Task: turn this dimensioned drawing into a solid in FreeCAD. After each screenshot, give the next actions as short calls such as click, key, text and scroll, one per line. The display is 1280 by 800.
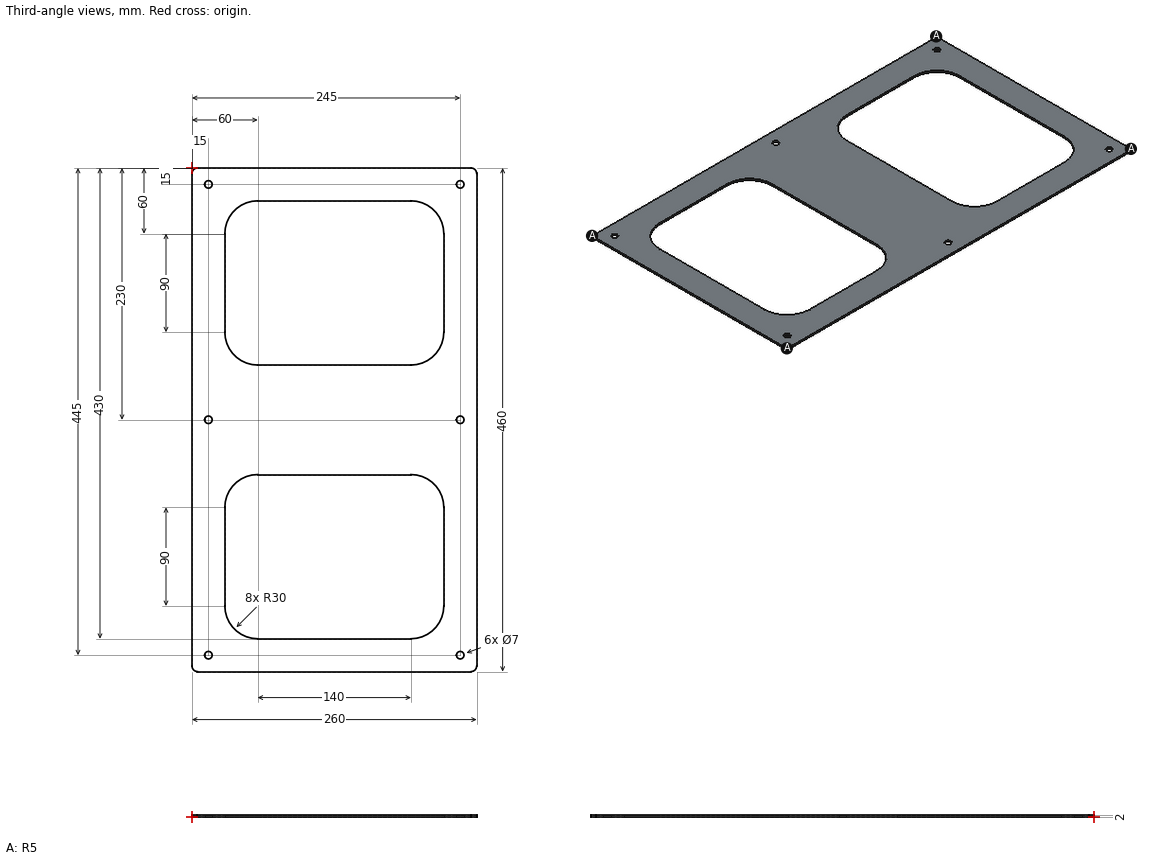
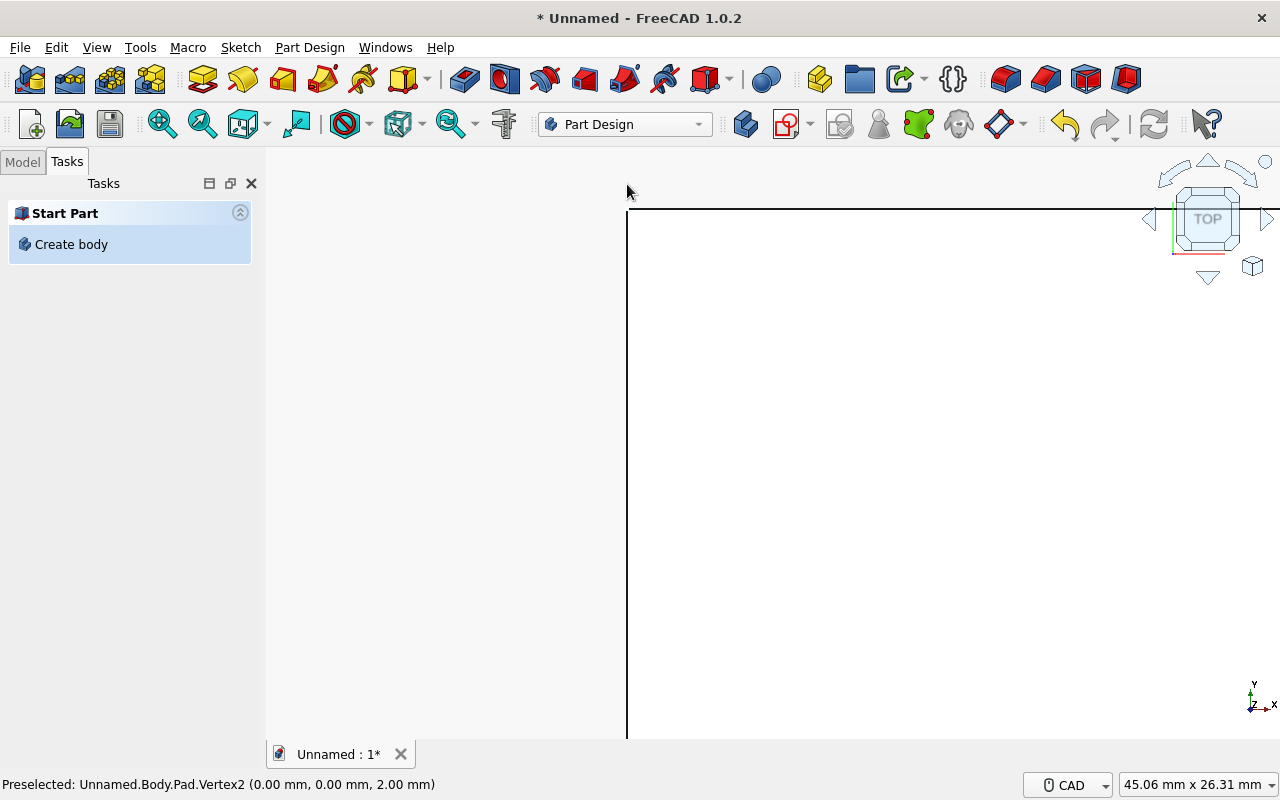
click(164, 124)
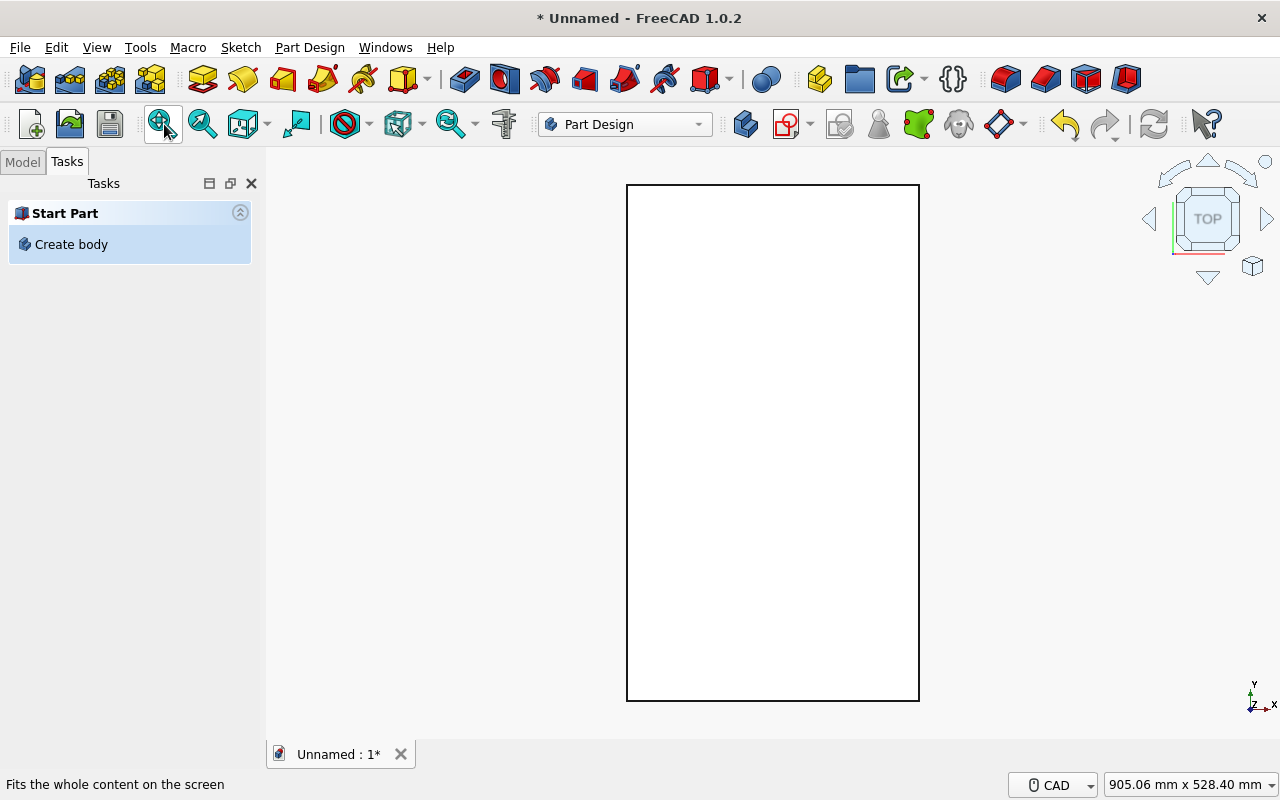
key(1)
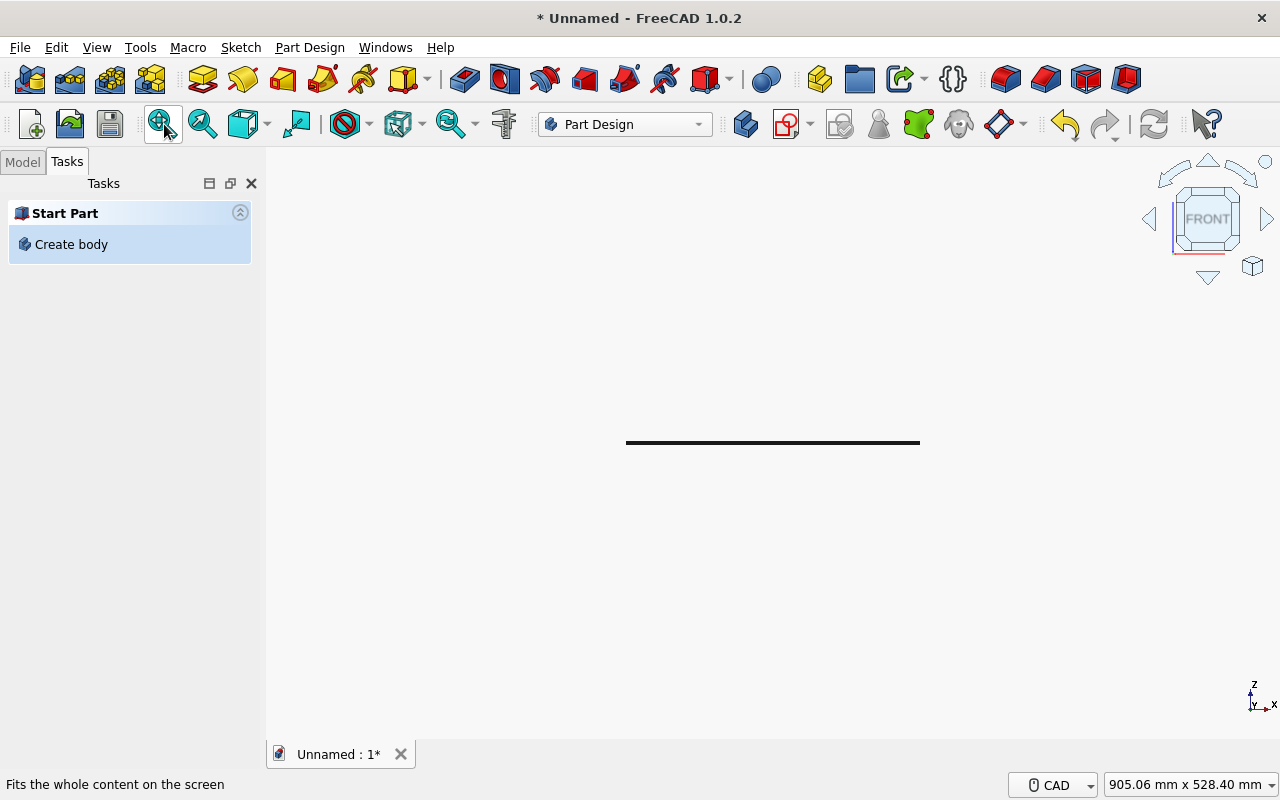
click(164, 124)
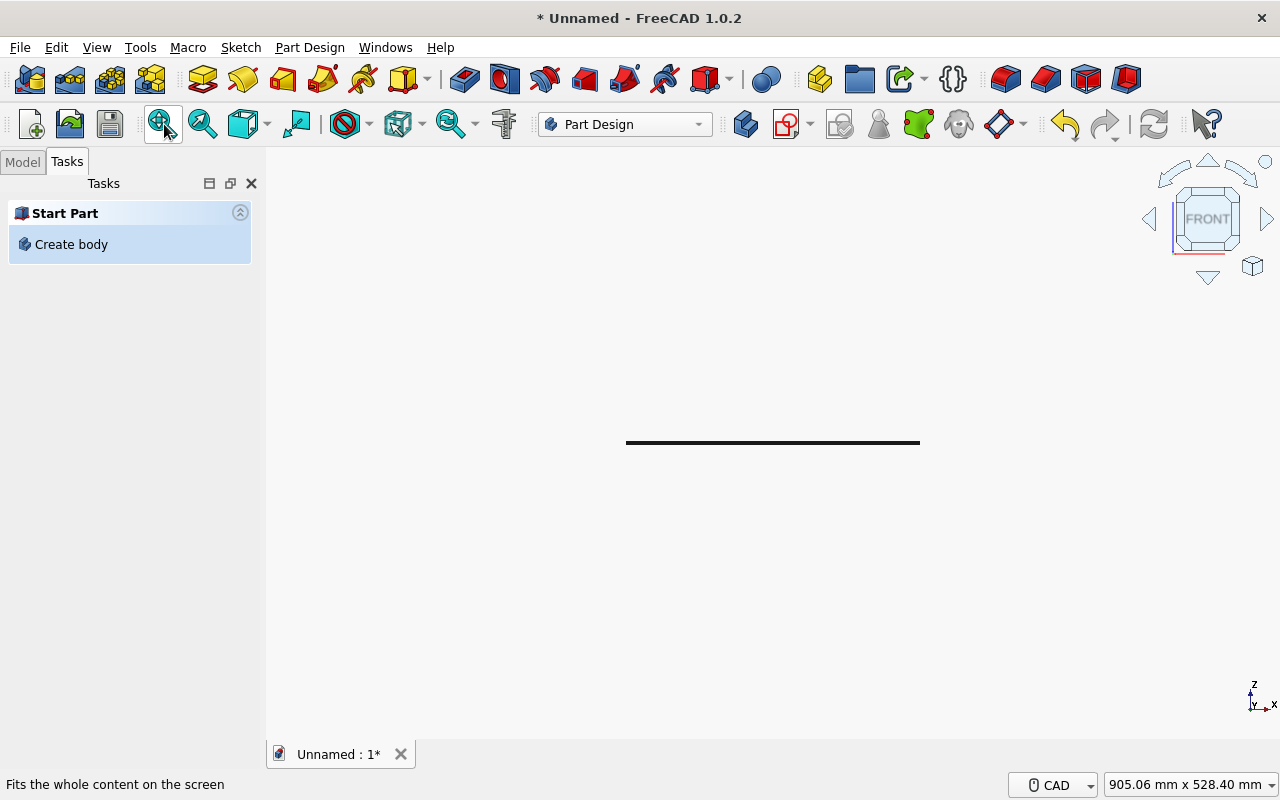
scroll(627, 442, up, 15)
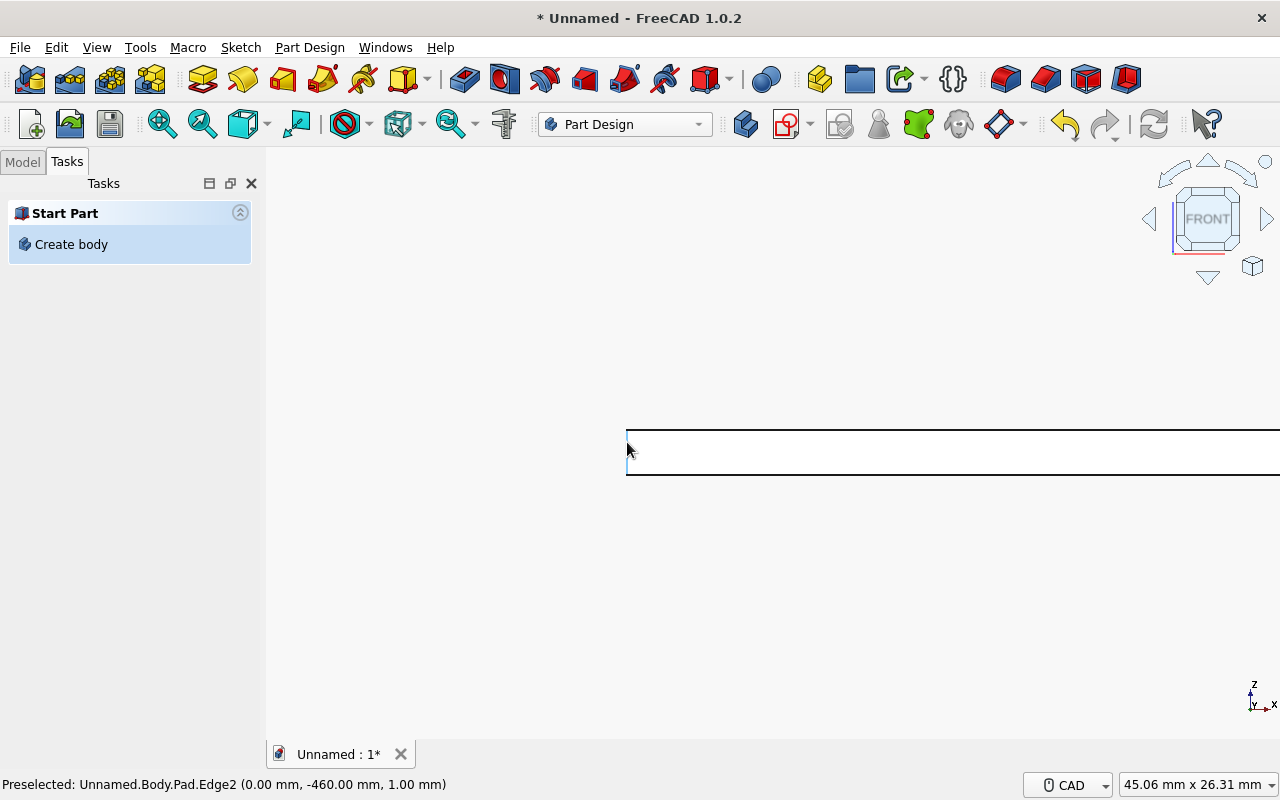
click(627, 452)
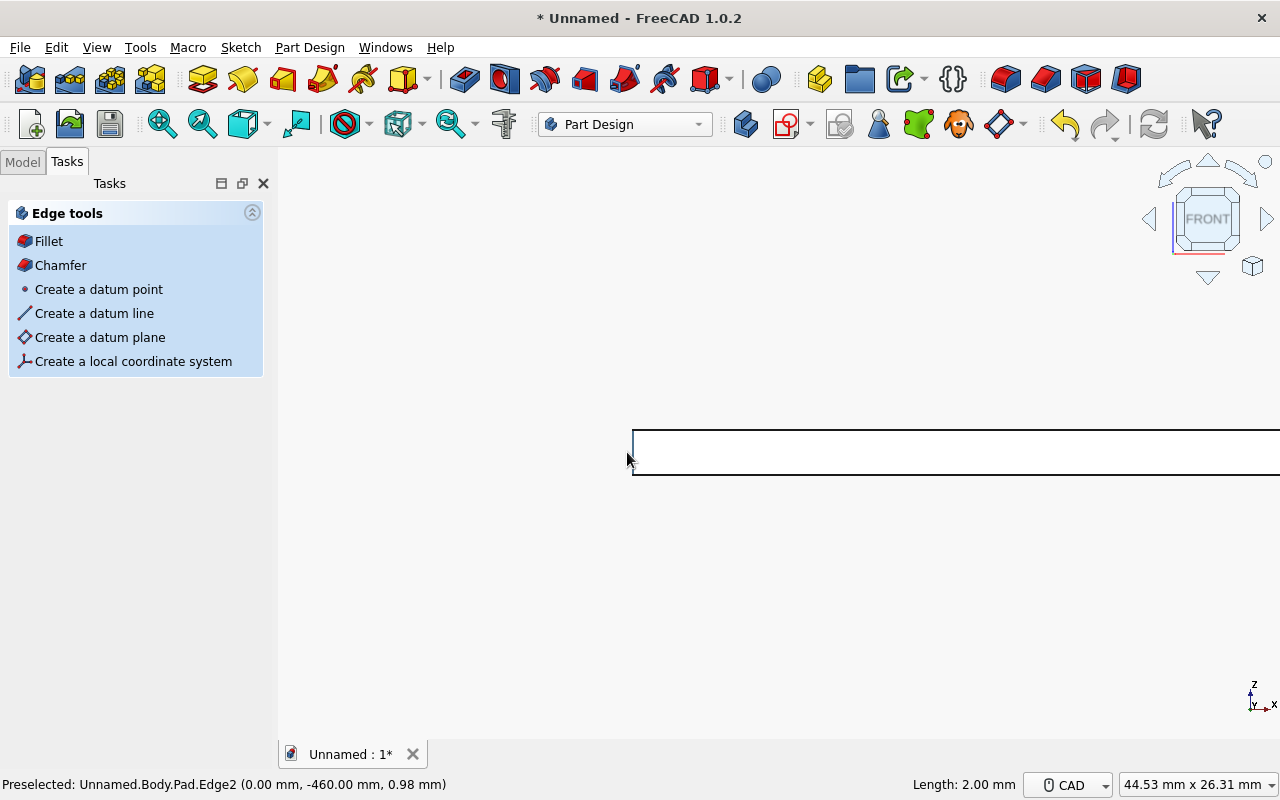
click(164, 124)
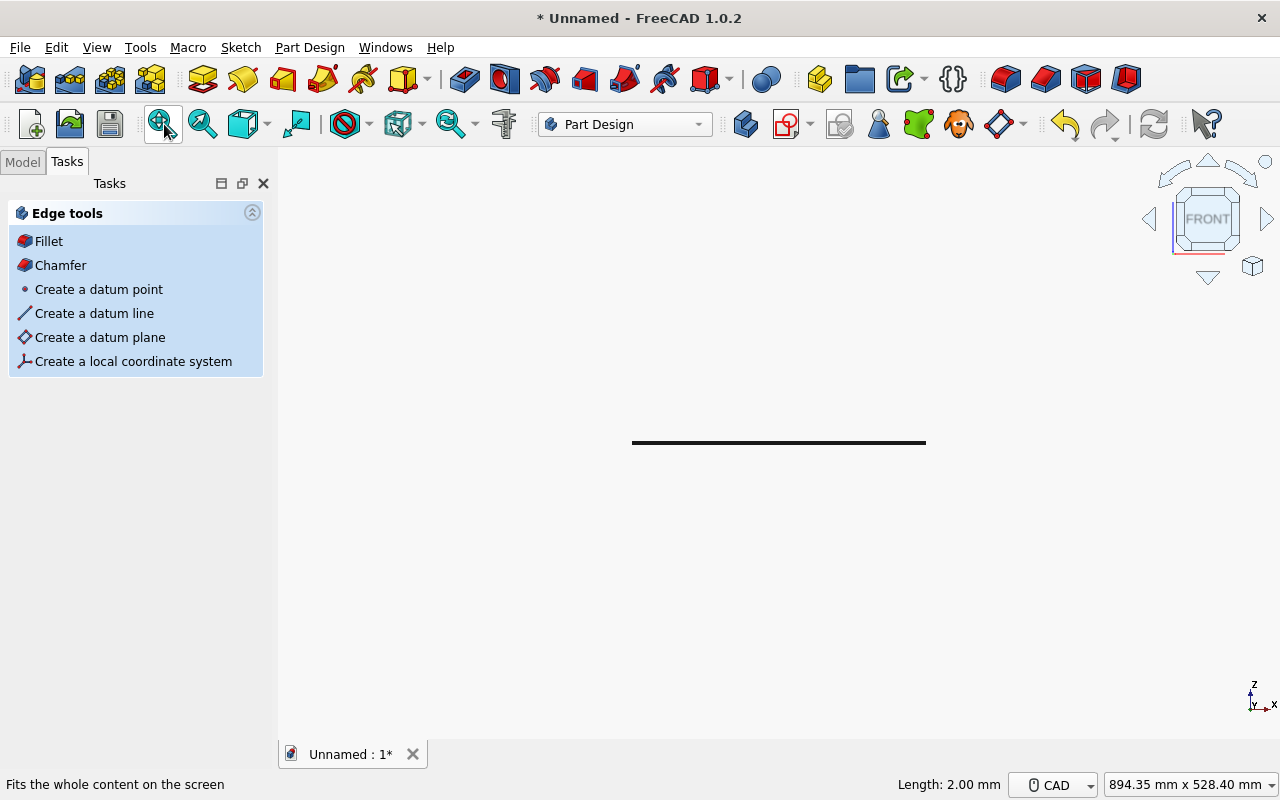
key(3)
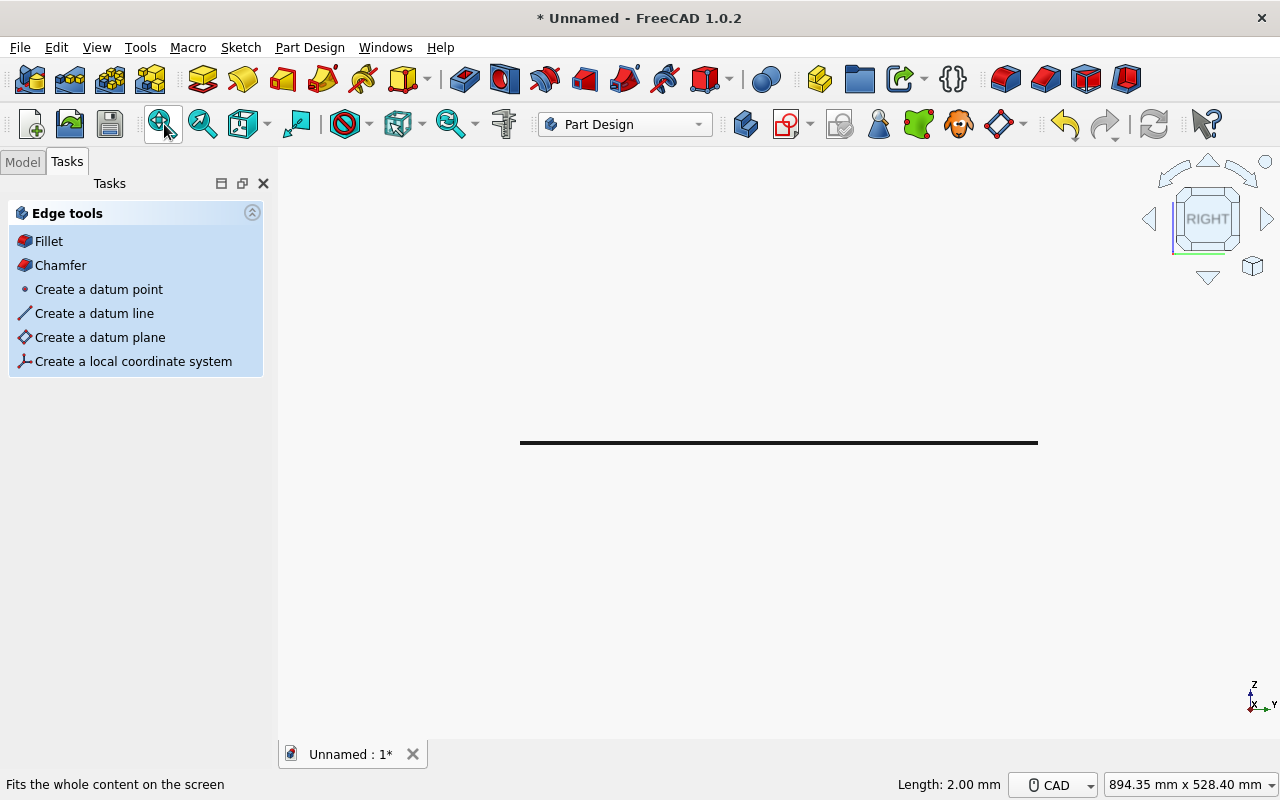
scroll(1037, 442, up, 15)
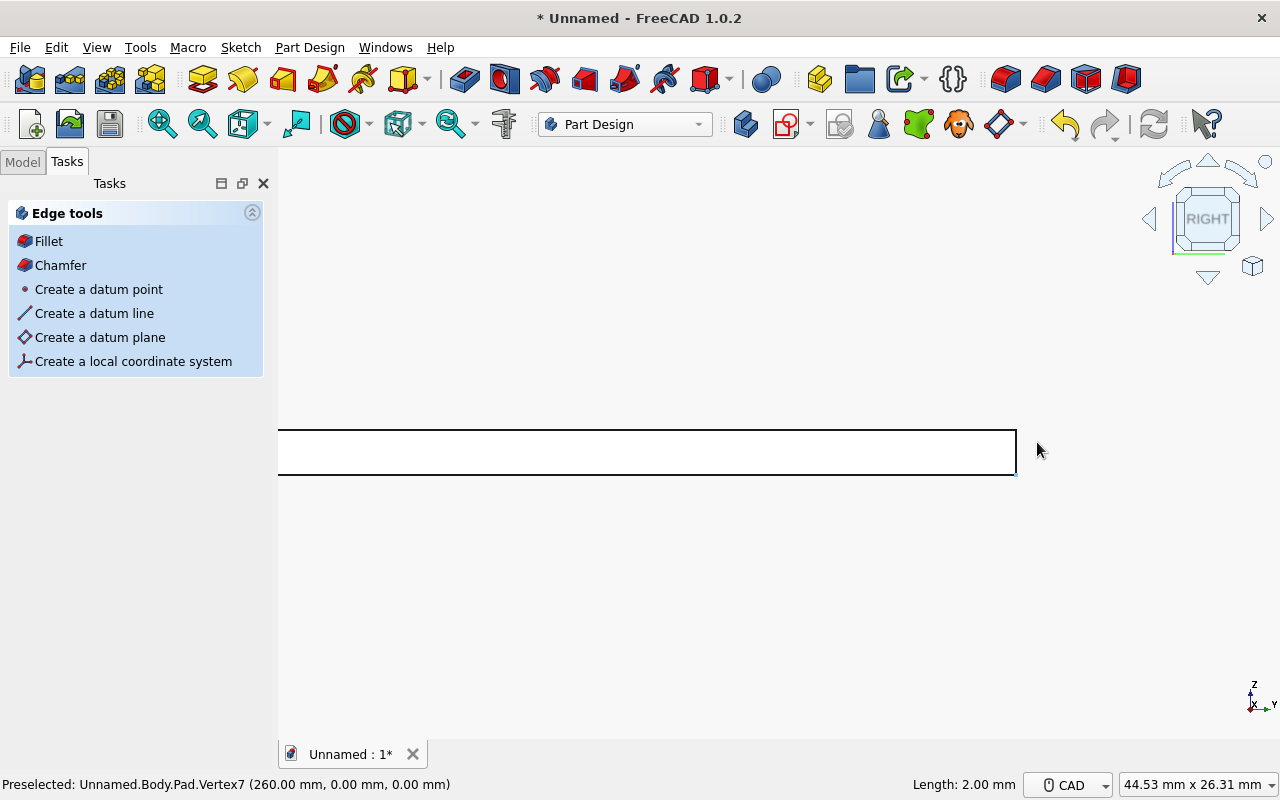
click(1016, 452, ctrl)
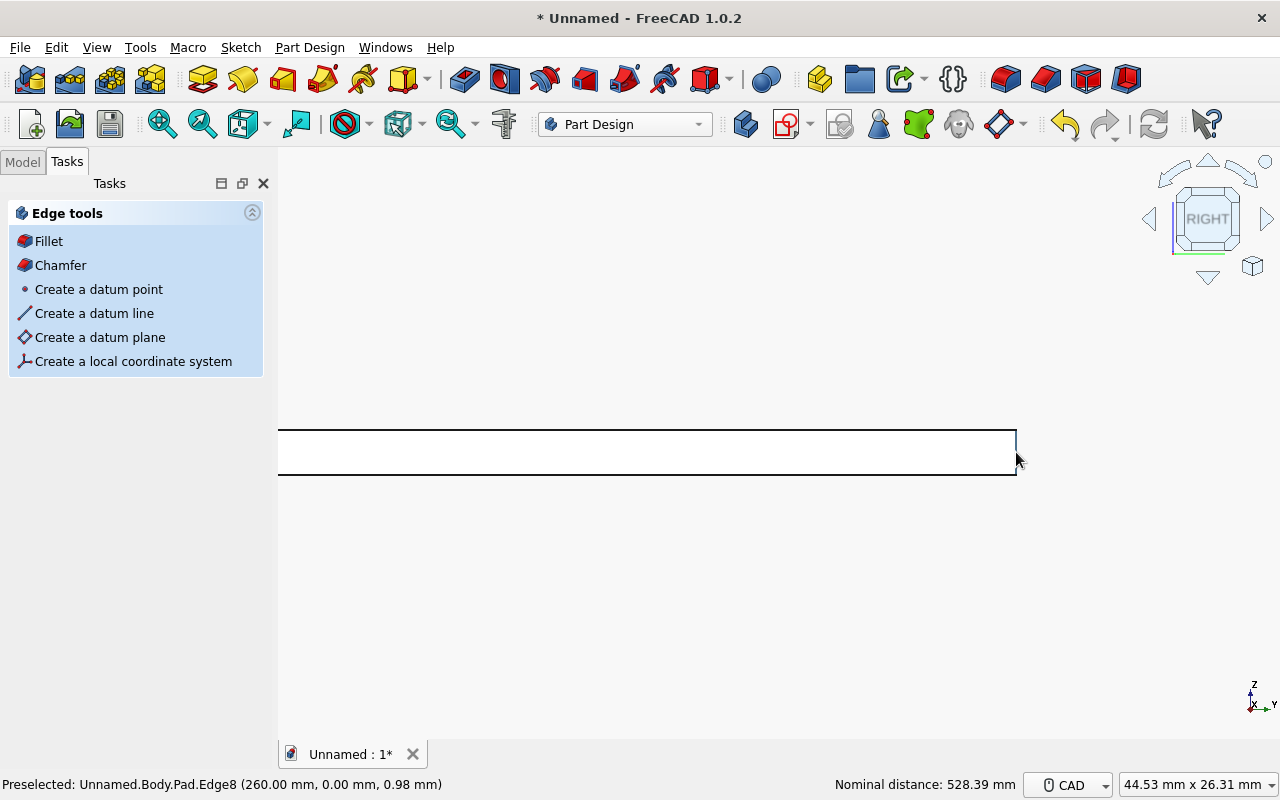
click(164, 124)